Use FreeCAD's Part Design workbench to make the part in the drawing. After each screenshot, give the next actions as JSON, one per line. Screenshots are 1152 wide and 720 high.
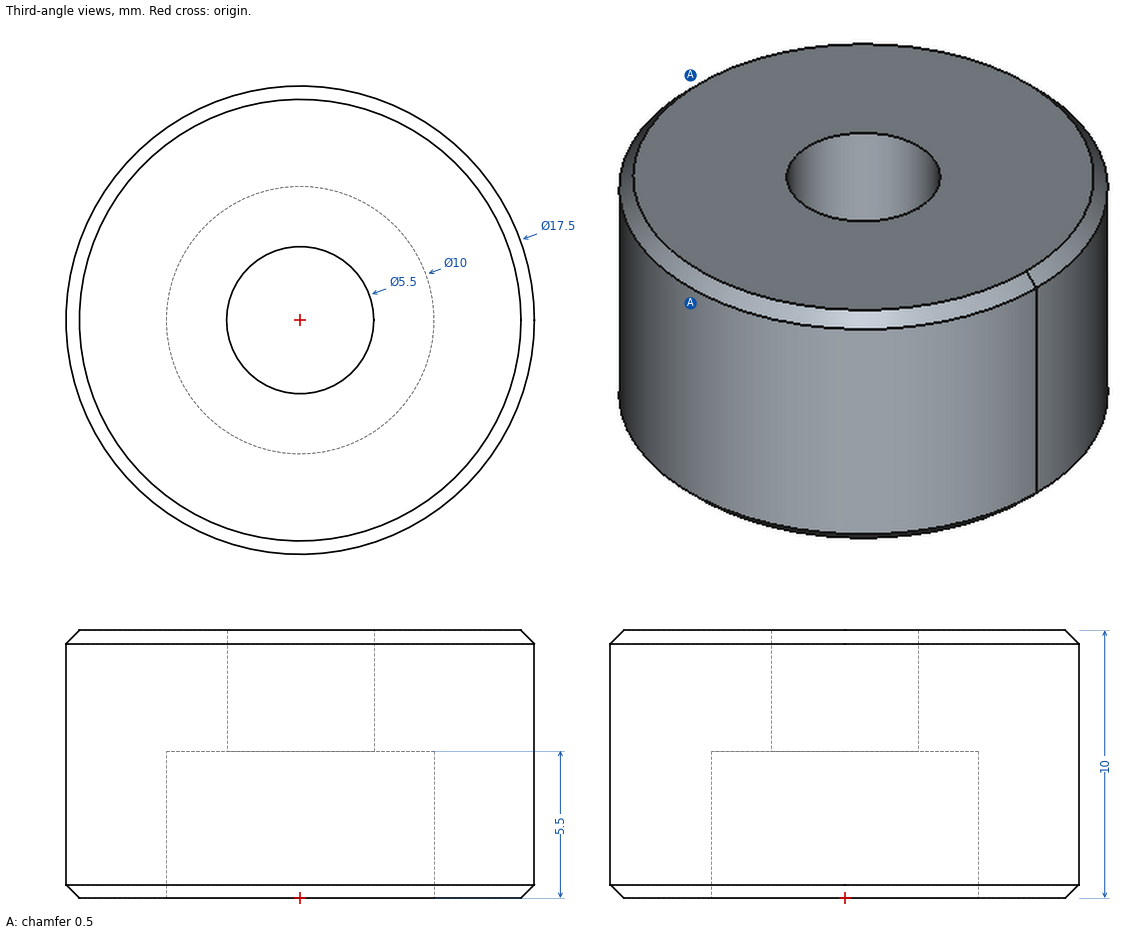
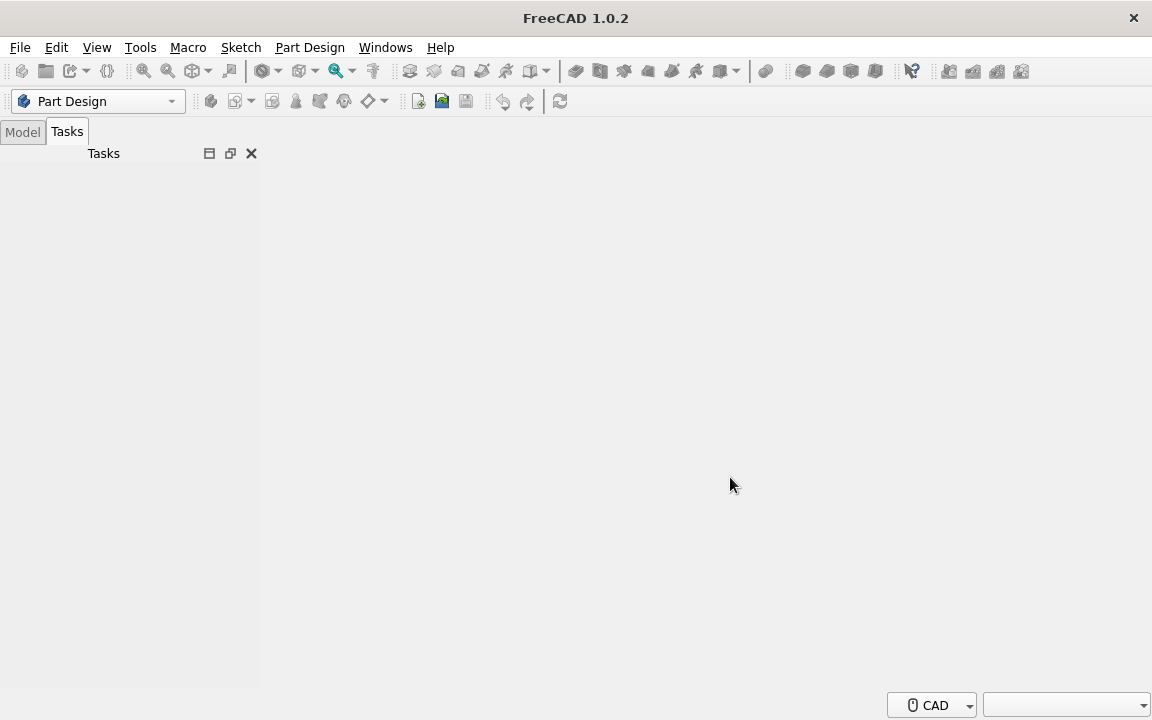
{"action": "left_click", "coordinate": [418, 102]}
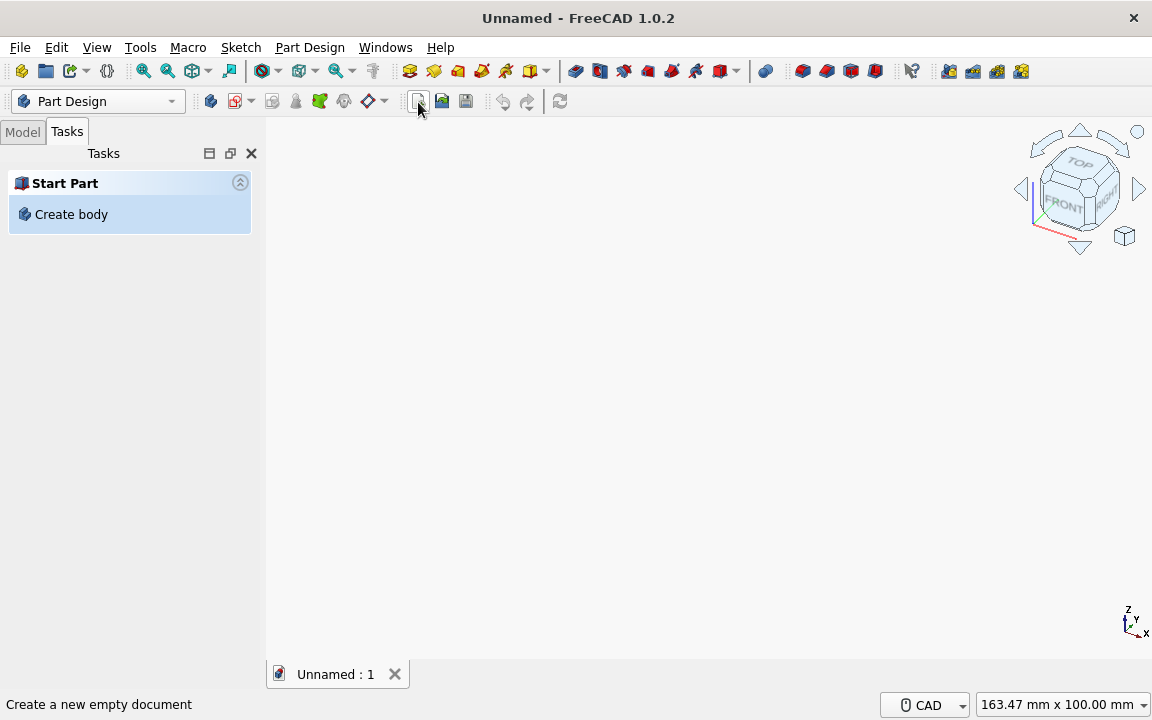
{"action": "left_click", "coordinate": [236, 102]}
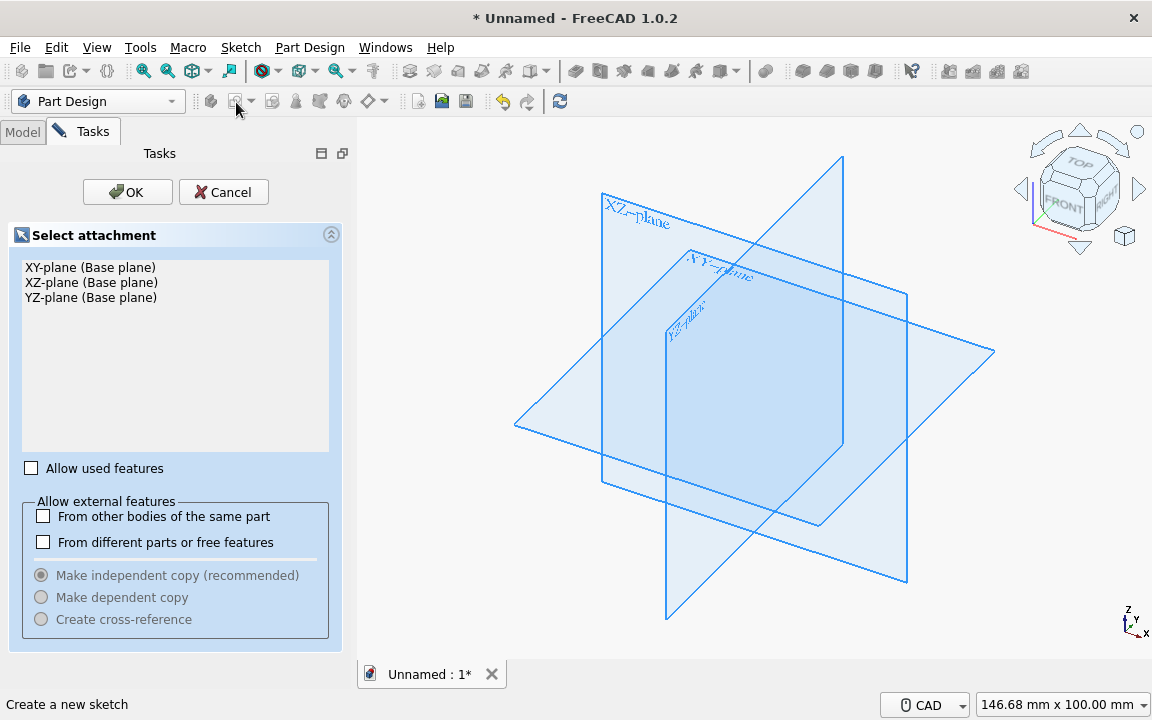
{"action": "left_click", "coordinate": [82, 268]}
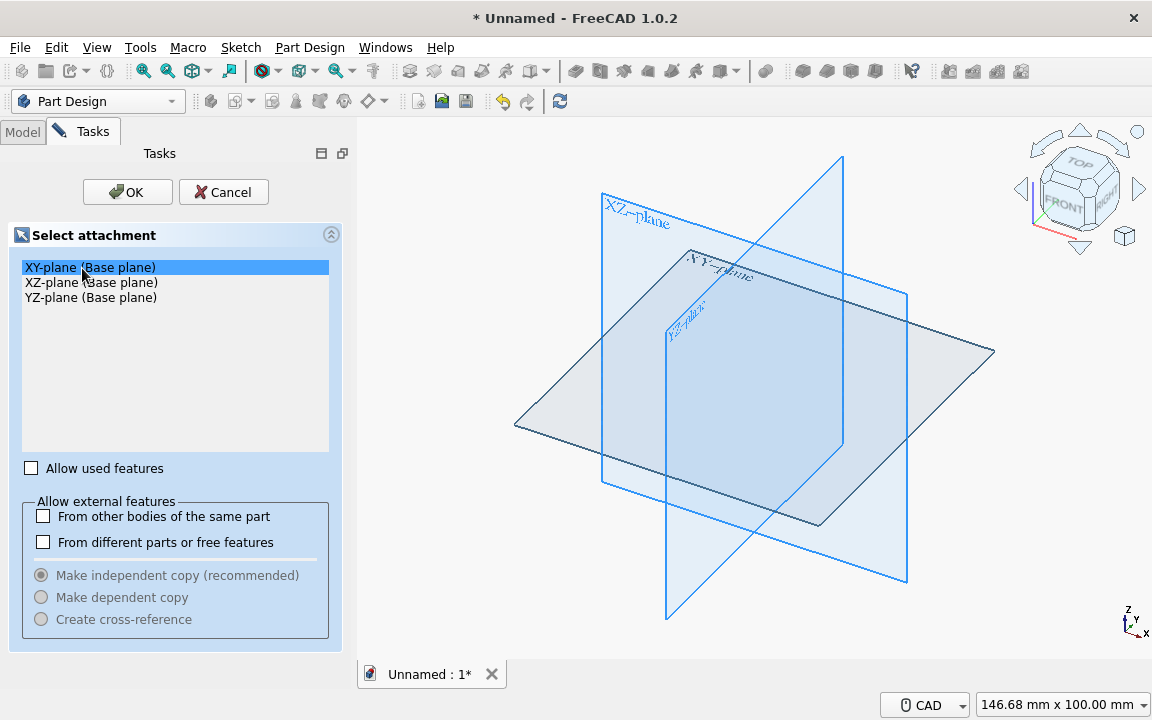
{"action": "left_click", "coordinate": [128, 192]}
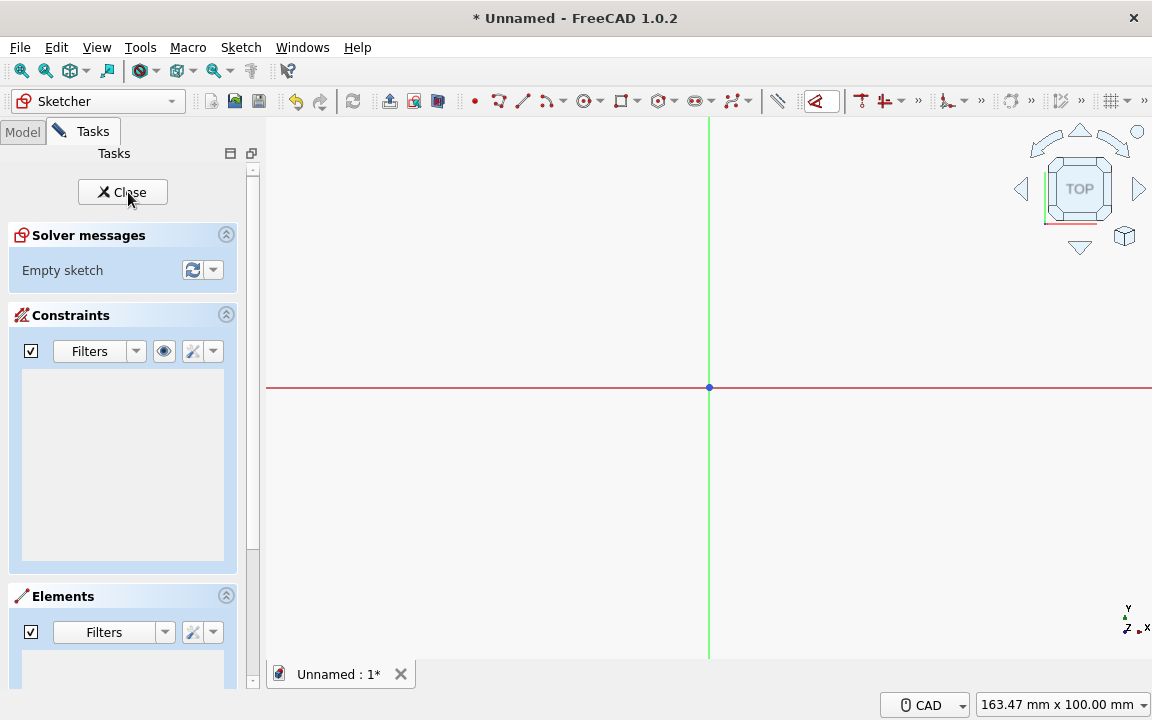
{"action": "scroll", "coordinate": [739, 388], "scroll_direction": "up", "scroll_amount": 6}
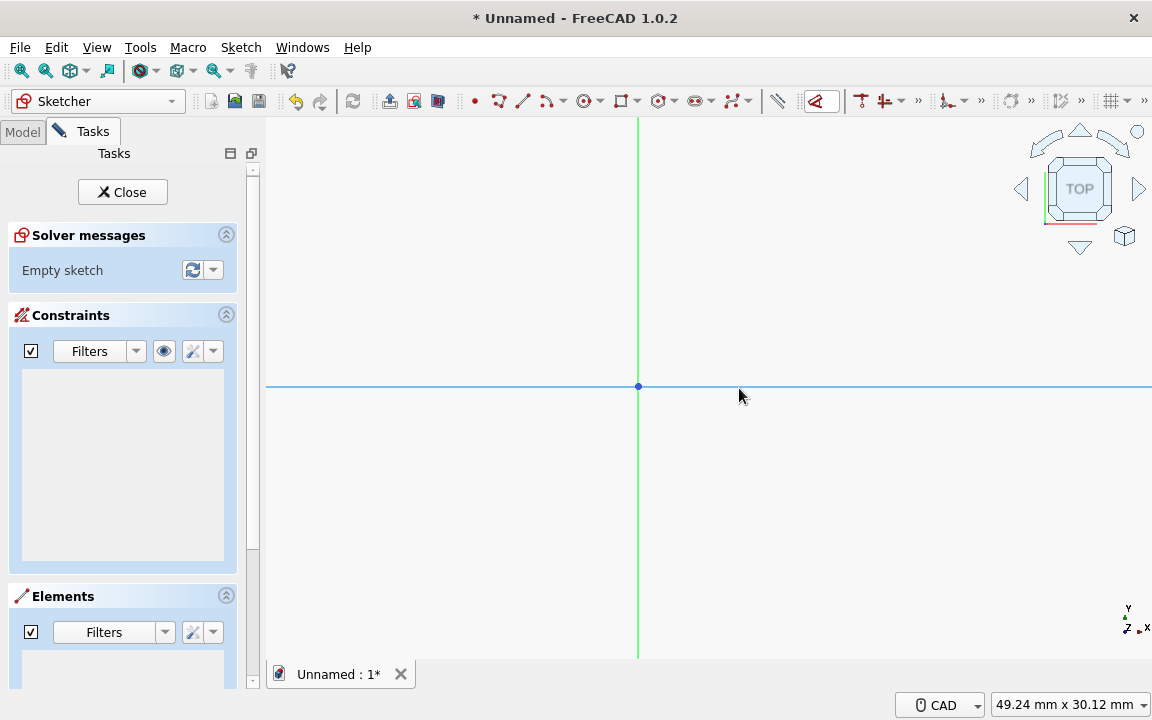
{"action": "key", "text": "g c"}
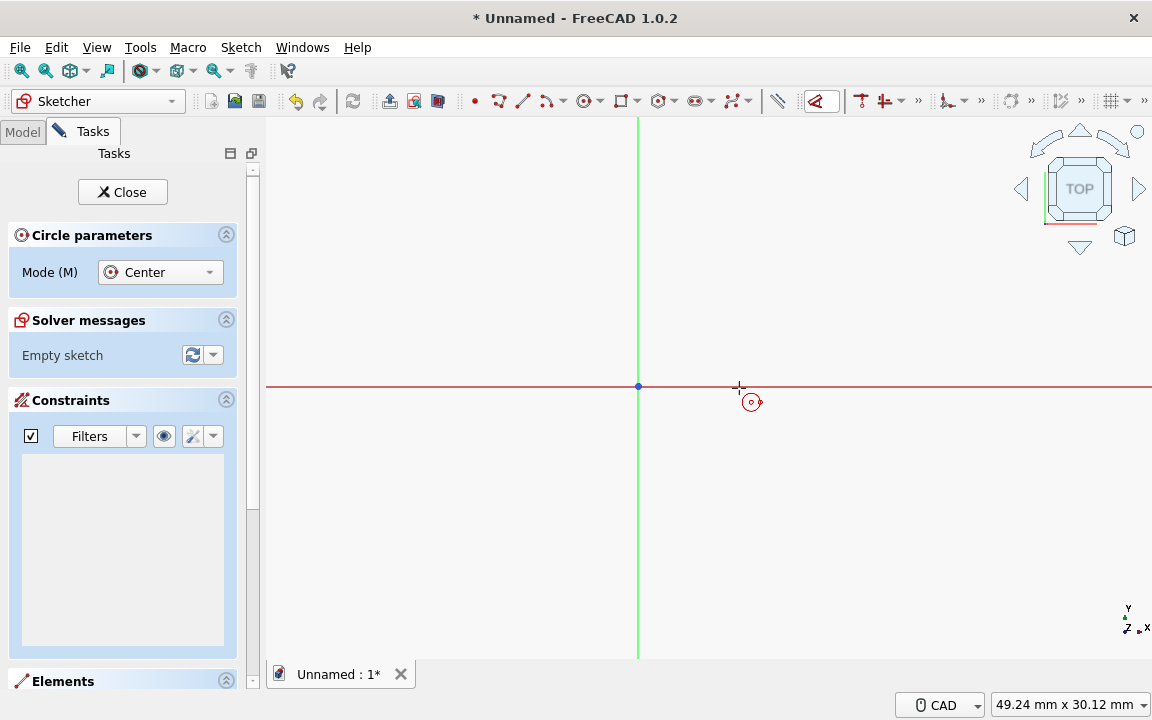
{"action": "left_click", "coordinate": [638, 387]}
{"action": "left_click", "coordinate": [749, 275]}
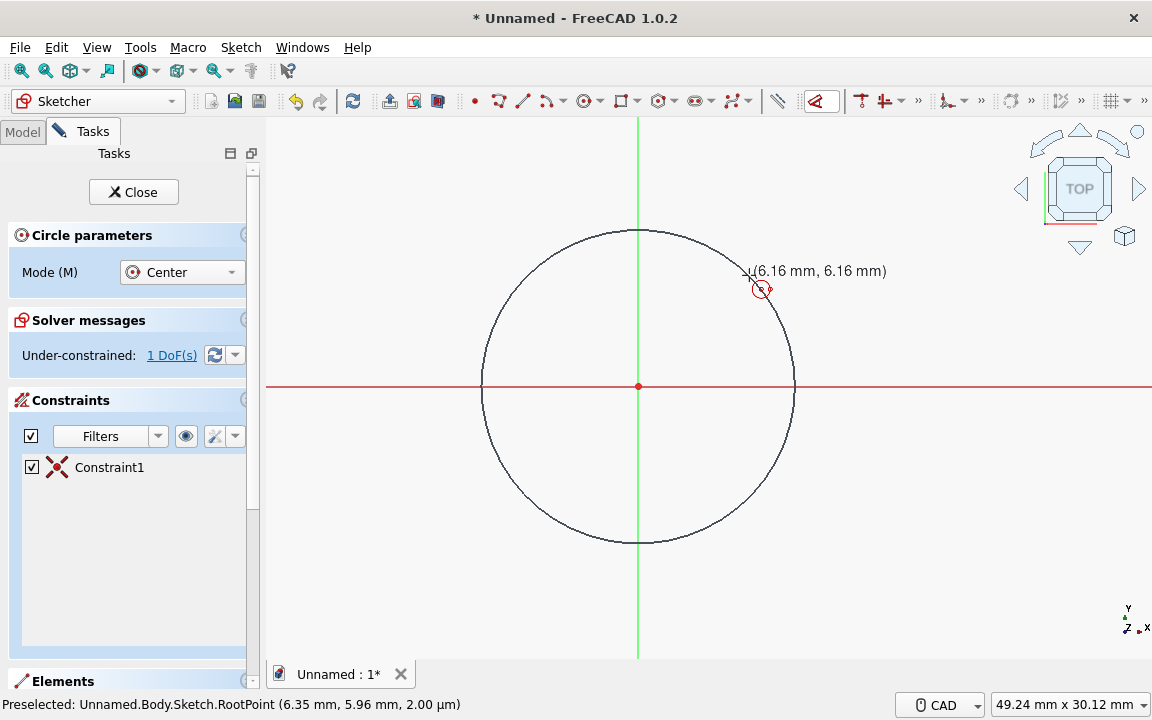
{"action": "left_click", "coordinate": [638, 387]}
{"action": "left_click", "coordinate": [673, 352]}
{"action": "key", "text": "Escape"}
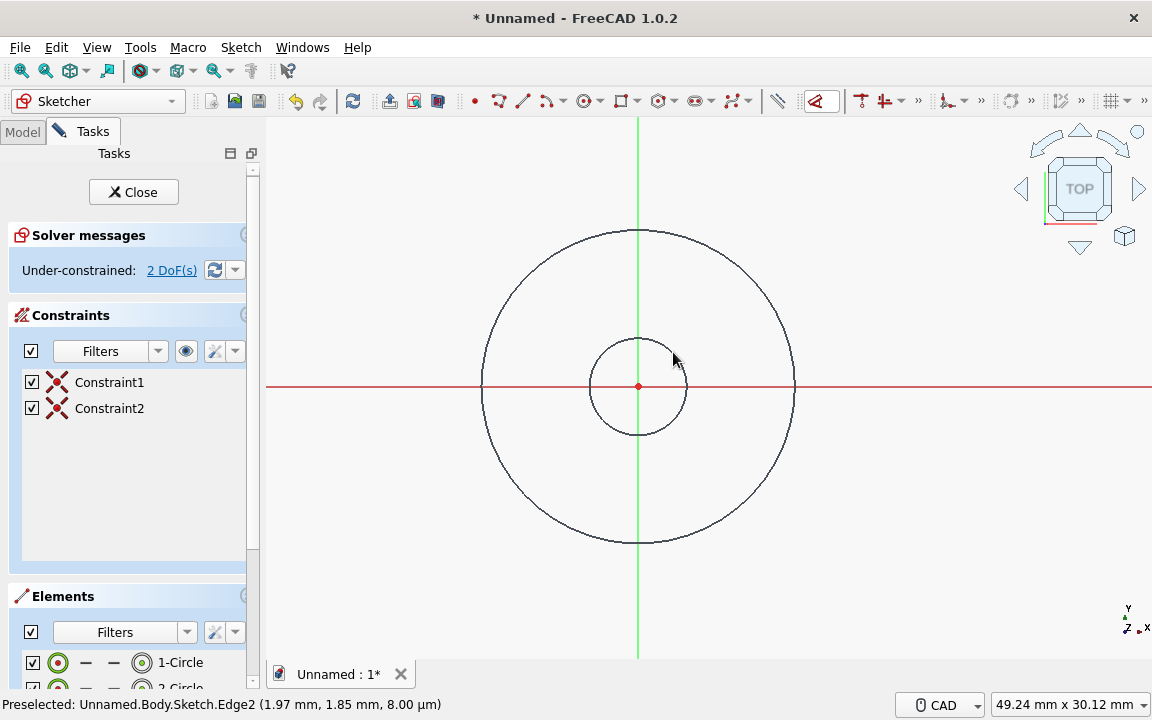
{"action": "key", "text": "d"}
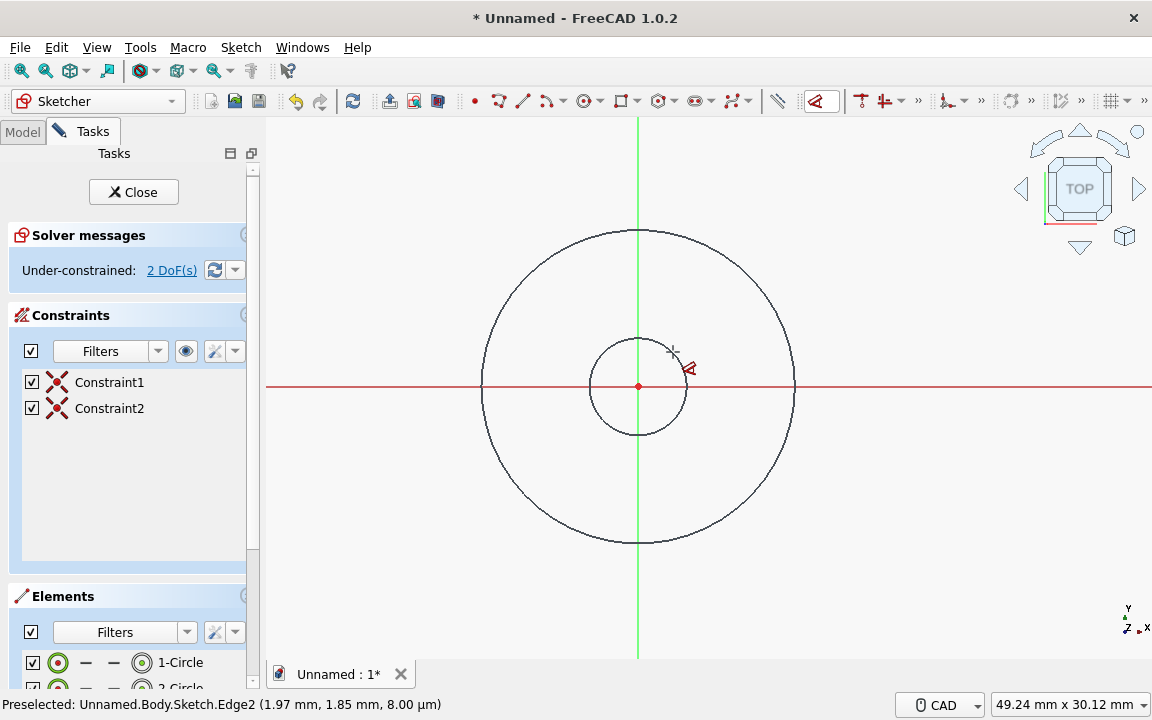
{"action": "left_click", "coordinate": [749, 276]}
{"action": "left_click", "coordinate": [772, 253]}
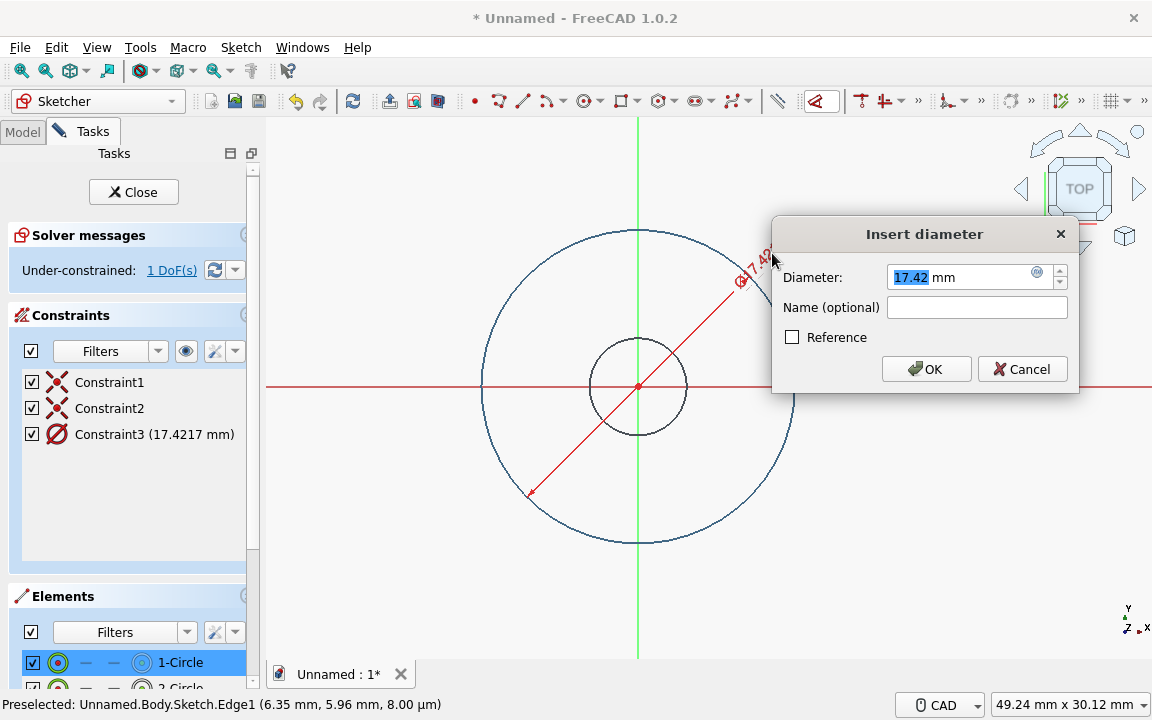
{"action": "type", "text": "17.5"}
{"action": "key", "text": "Return"}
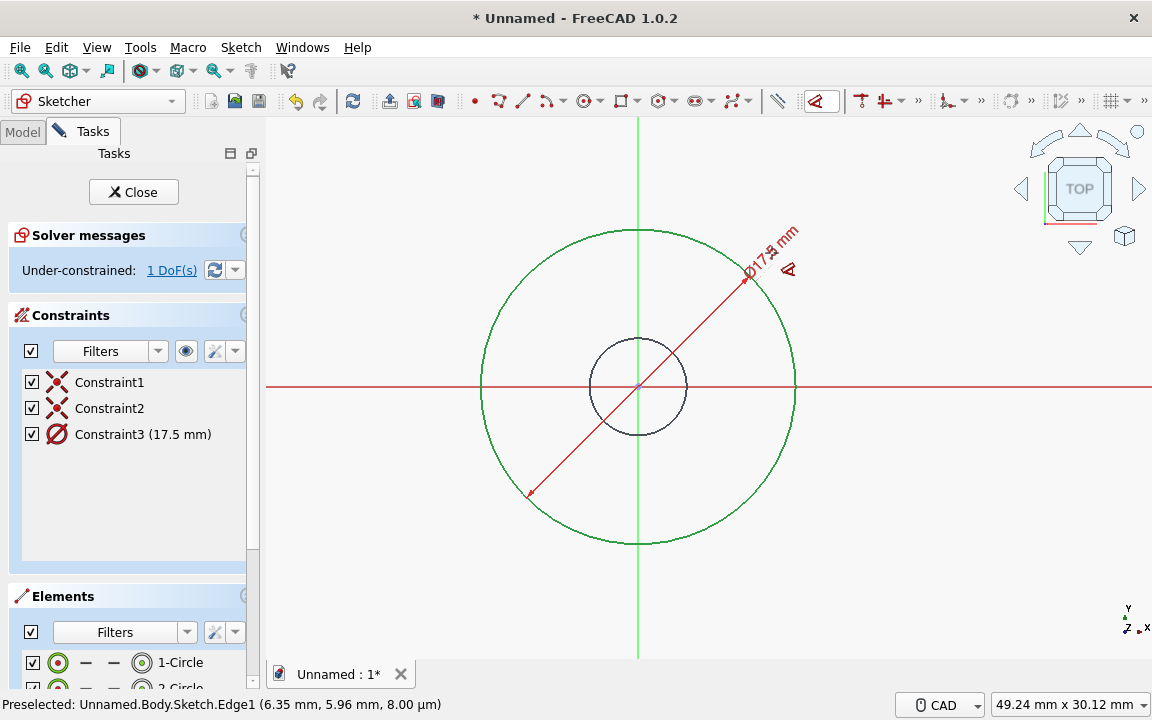
{"action": "left_click", "coordinate": [672, 352]}
{"action": "left_click", "coordinate": [694, 329]}